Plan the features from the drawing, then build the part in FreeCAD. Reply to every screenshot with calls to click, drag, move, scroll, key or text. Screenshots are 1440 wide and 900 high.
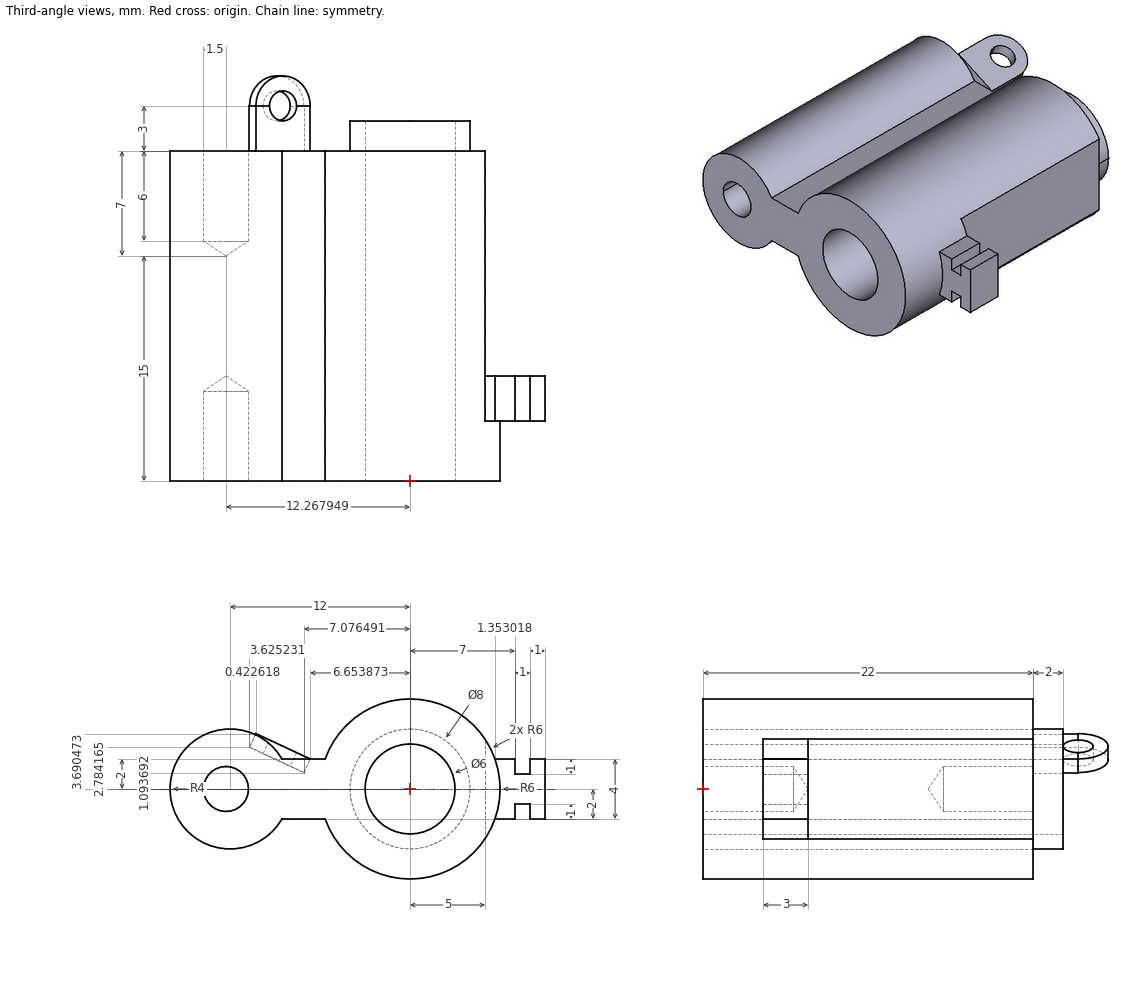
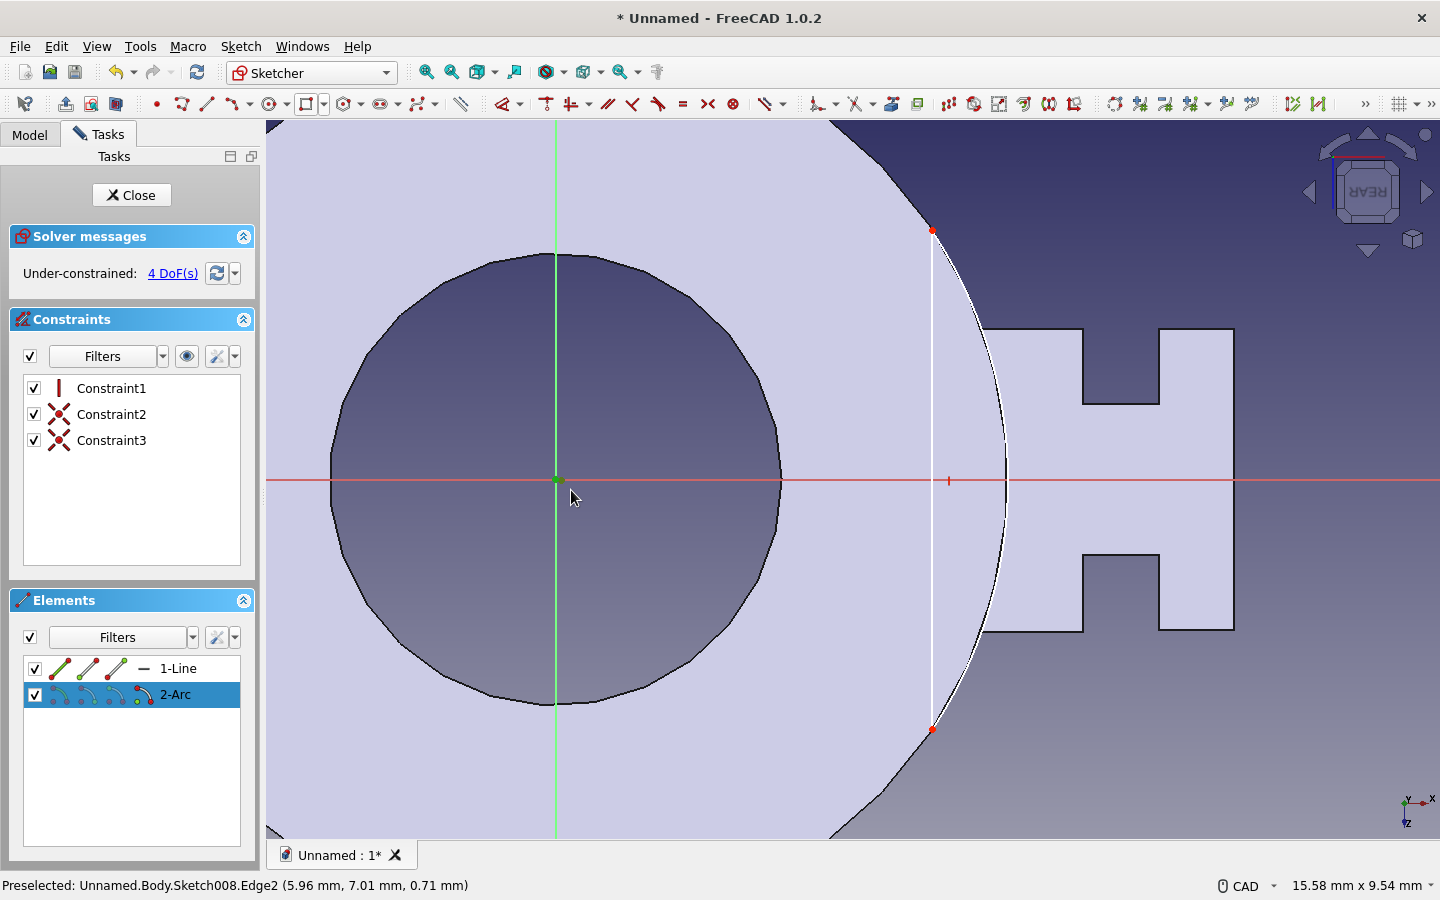
click(546, 104)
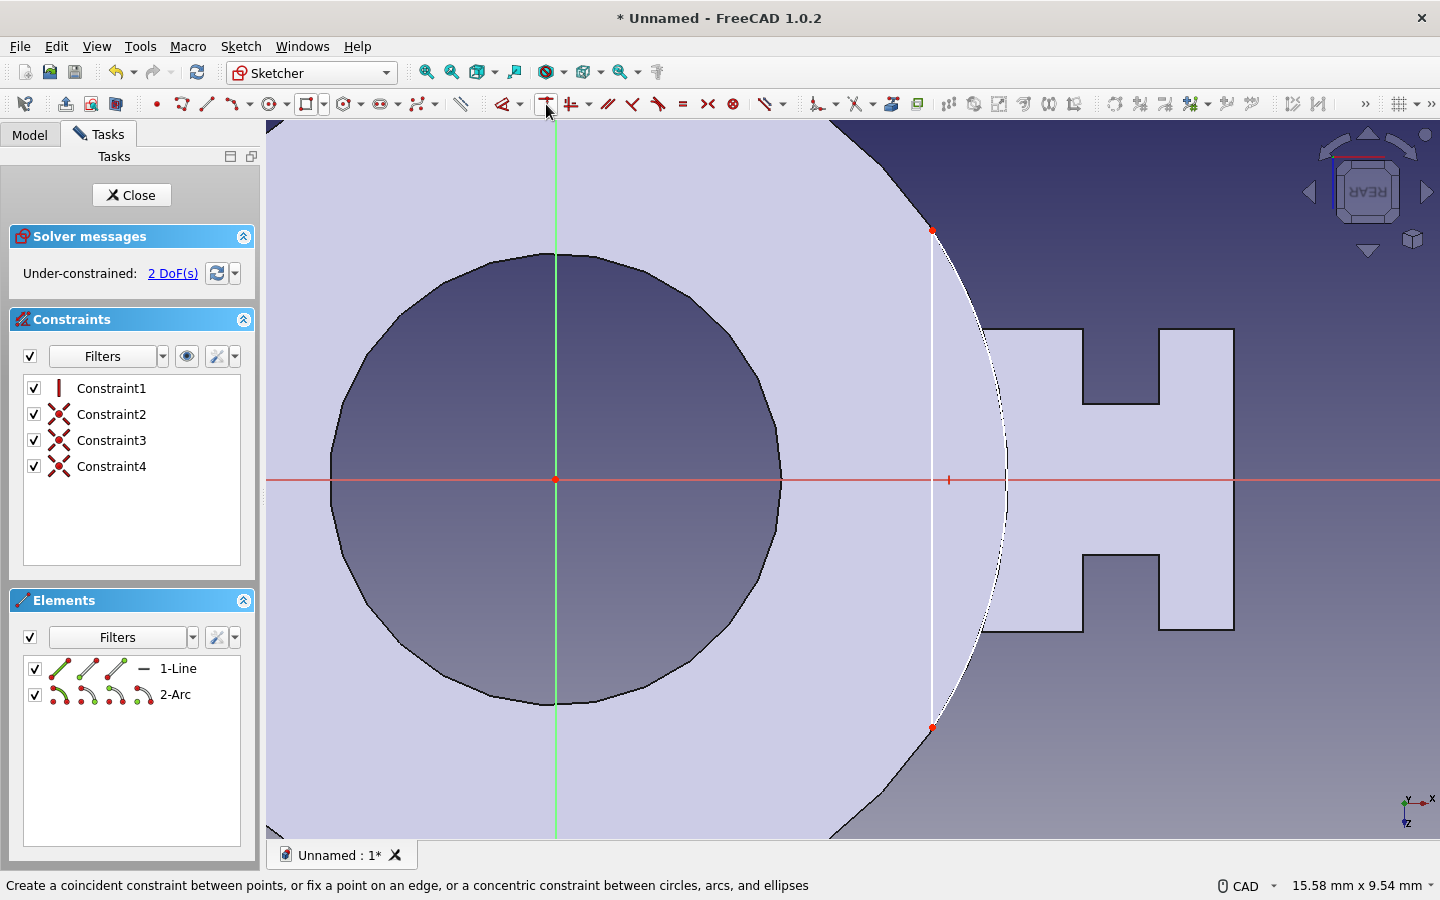
click(502, 104)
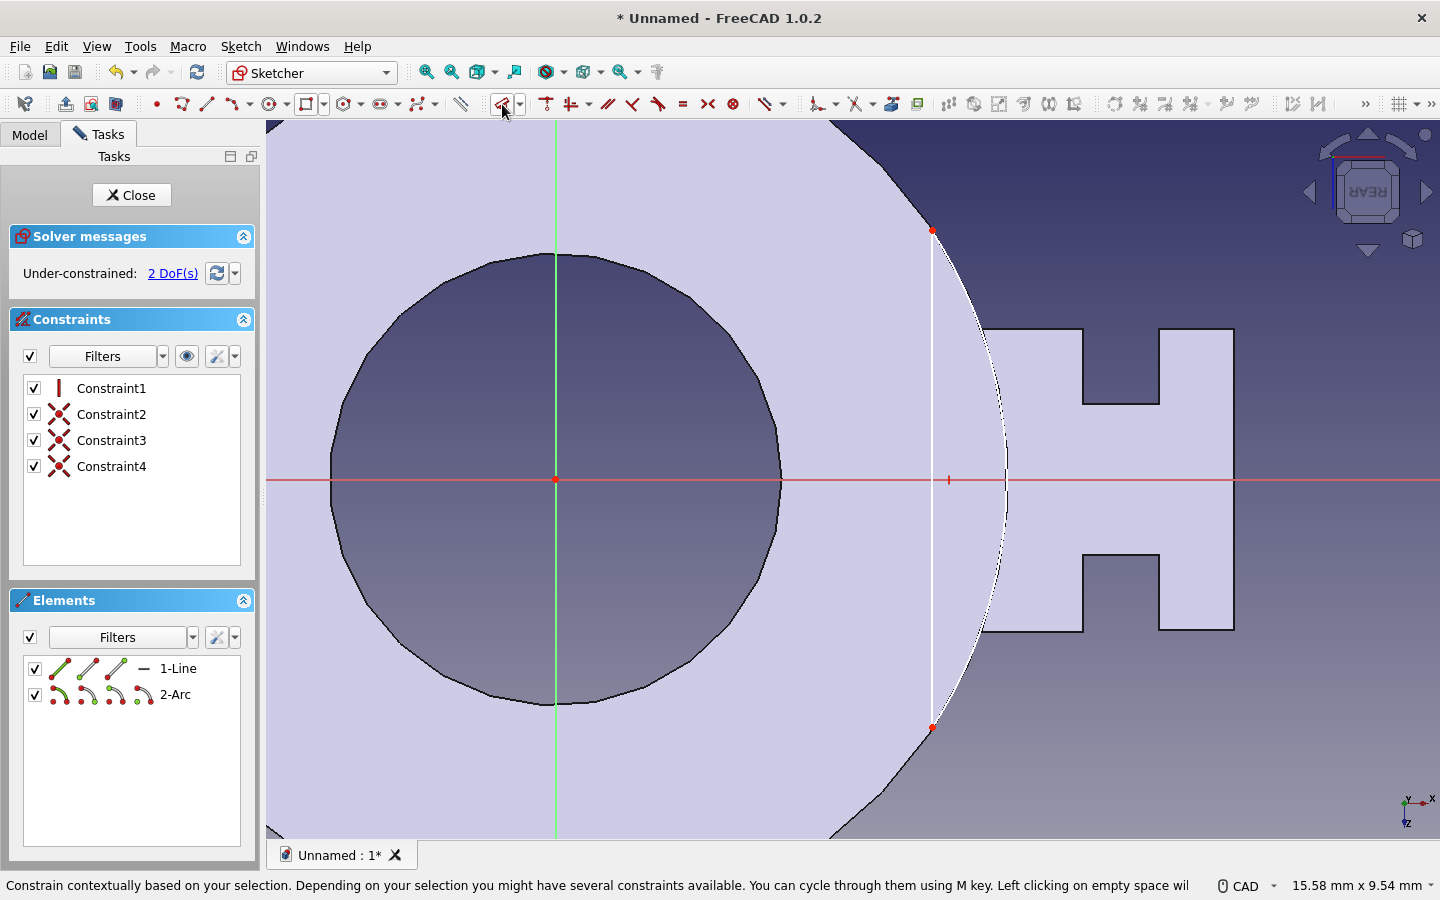
click(994, 584)
click(1025, 591)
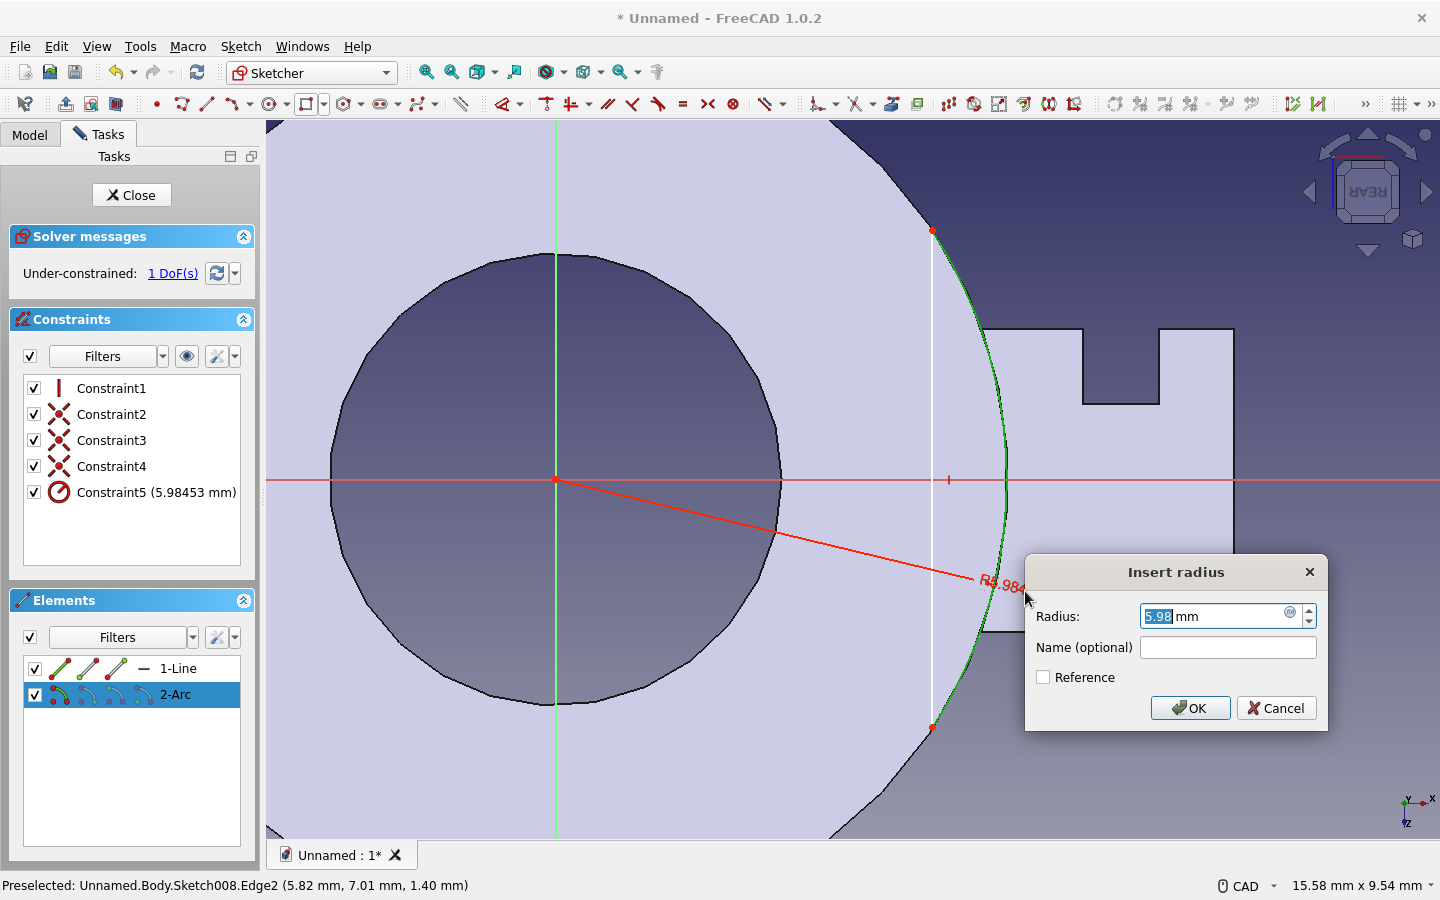
text(6)
key(Return)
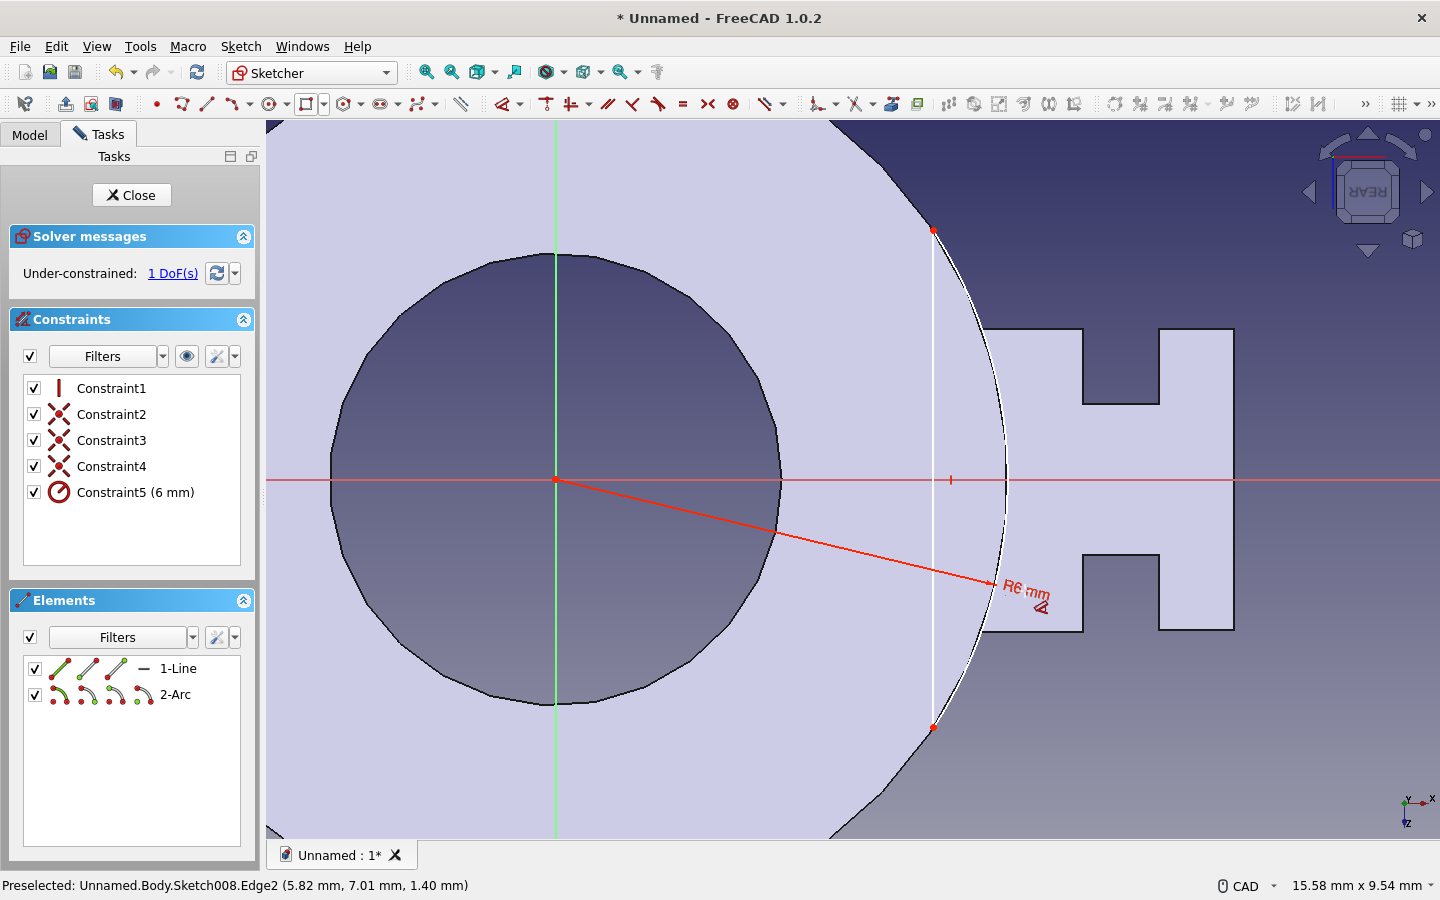
click(933, 231)
click(745, 197)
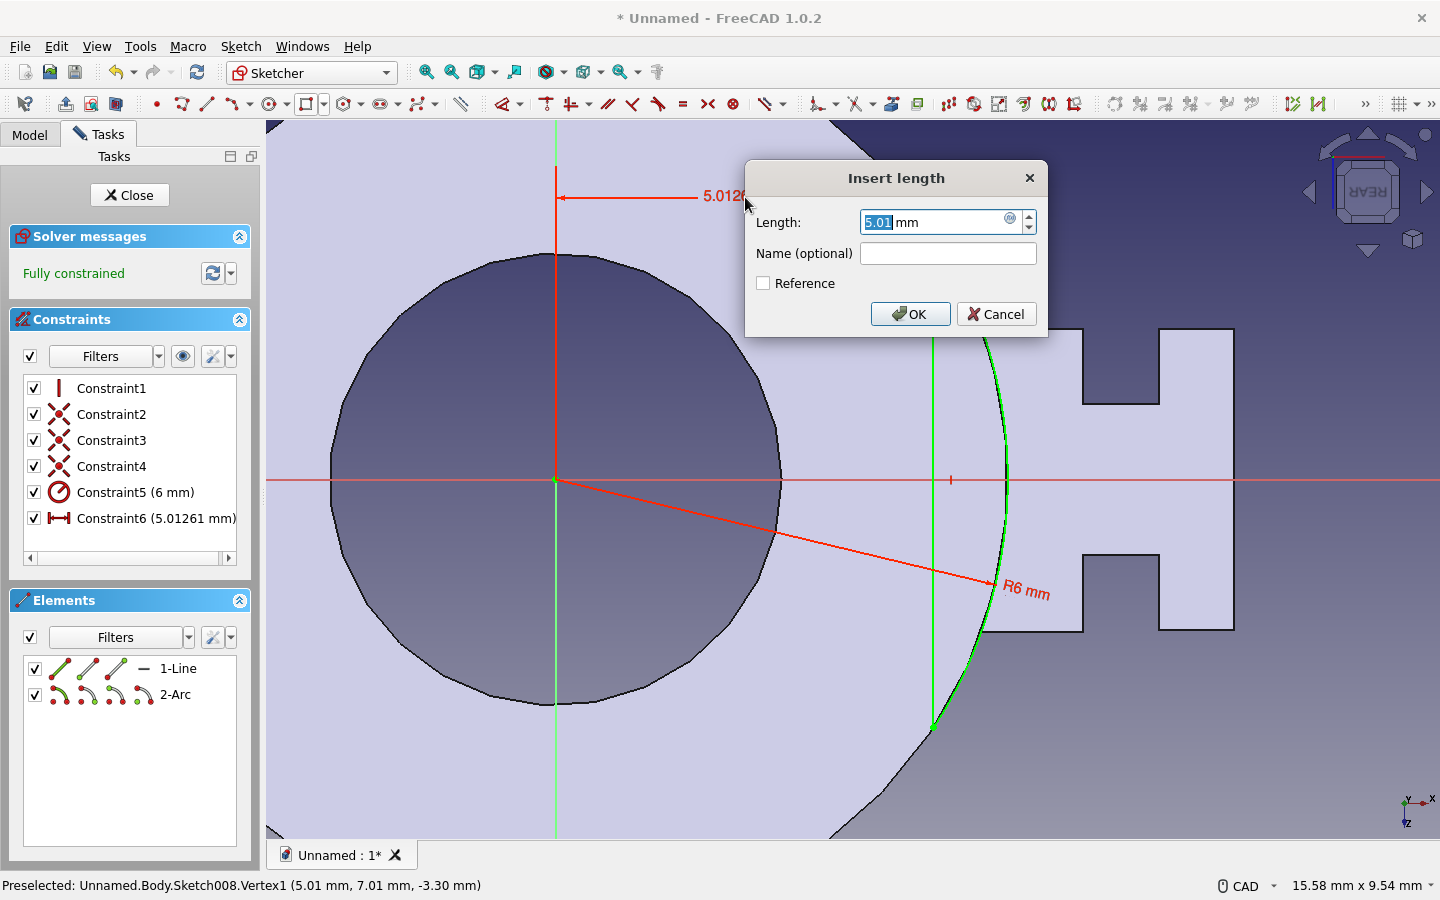
text(5)
key(Return)
key(Escape)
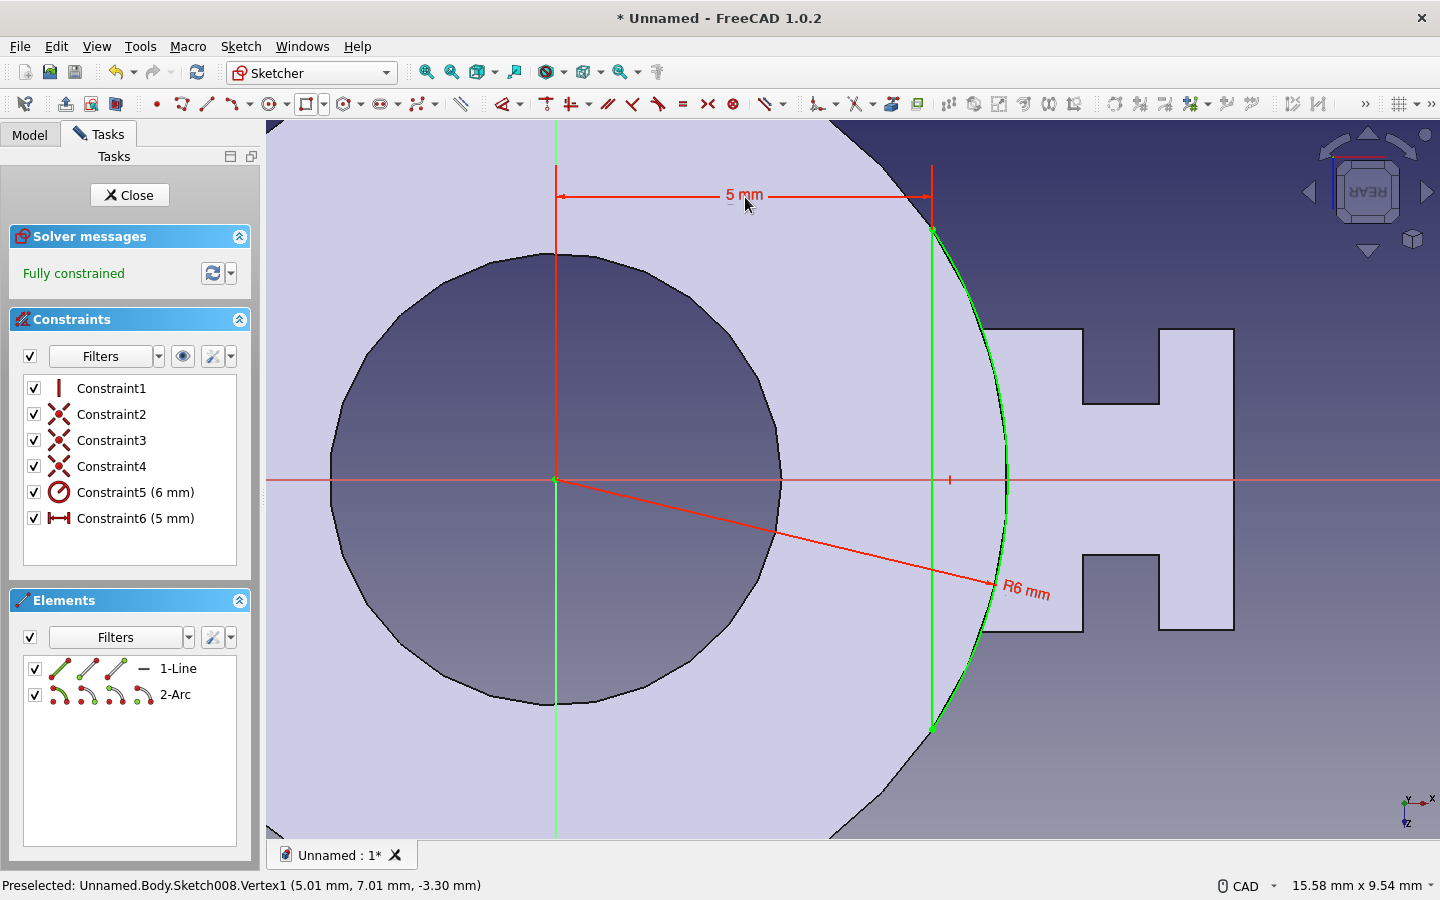
click(130, 195)